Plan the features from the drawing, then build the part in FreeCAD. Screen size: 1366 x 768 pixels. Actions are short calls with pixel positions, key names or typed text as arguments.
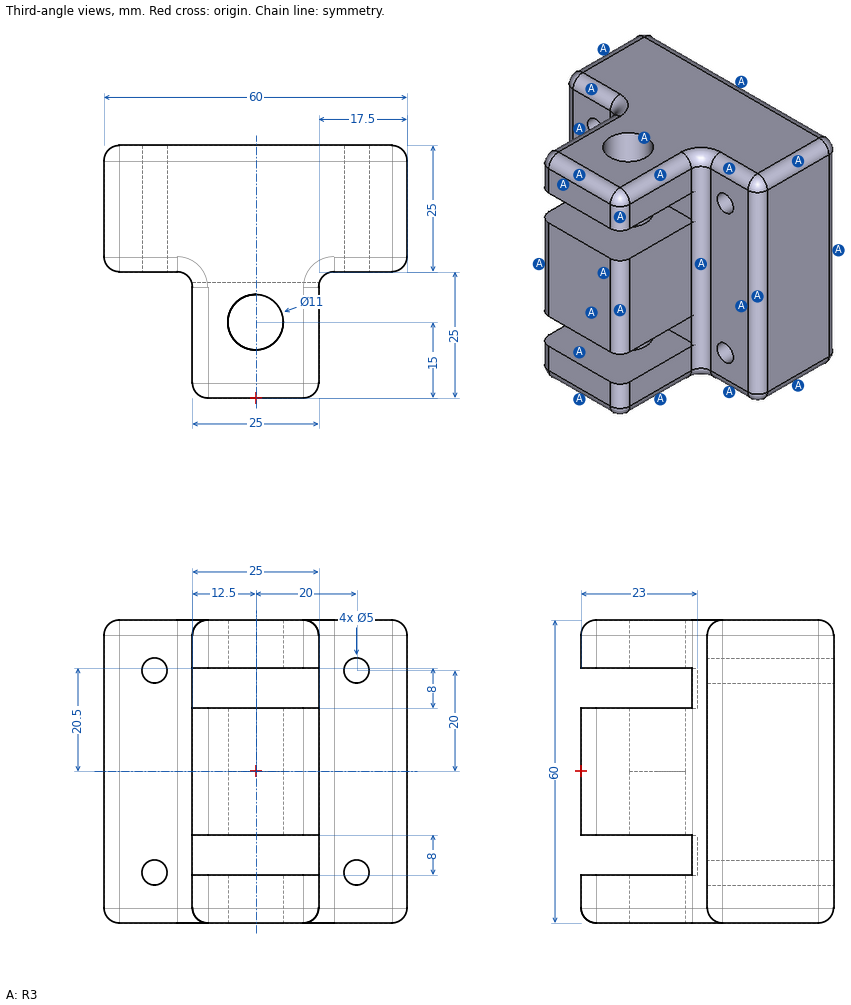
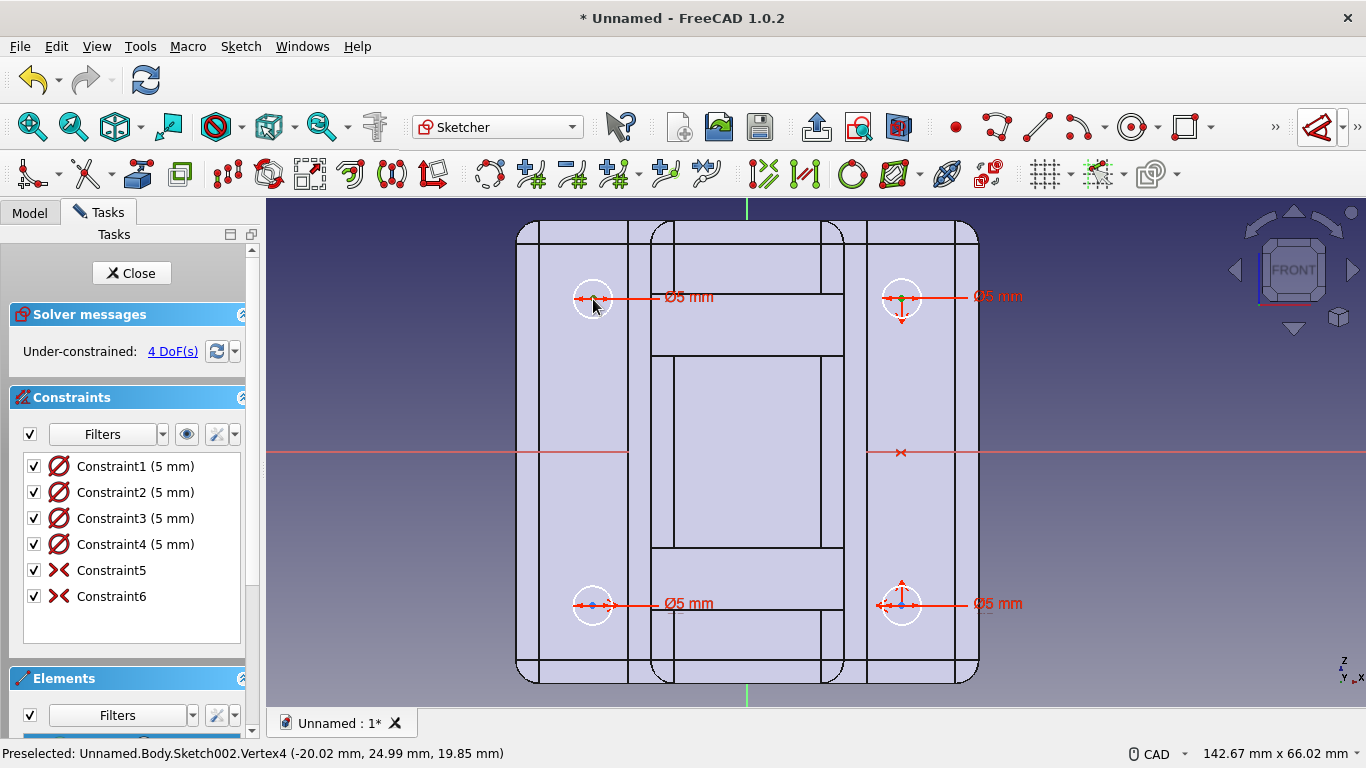
click(747, 647)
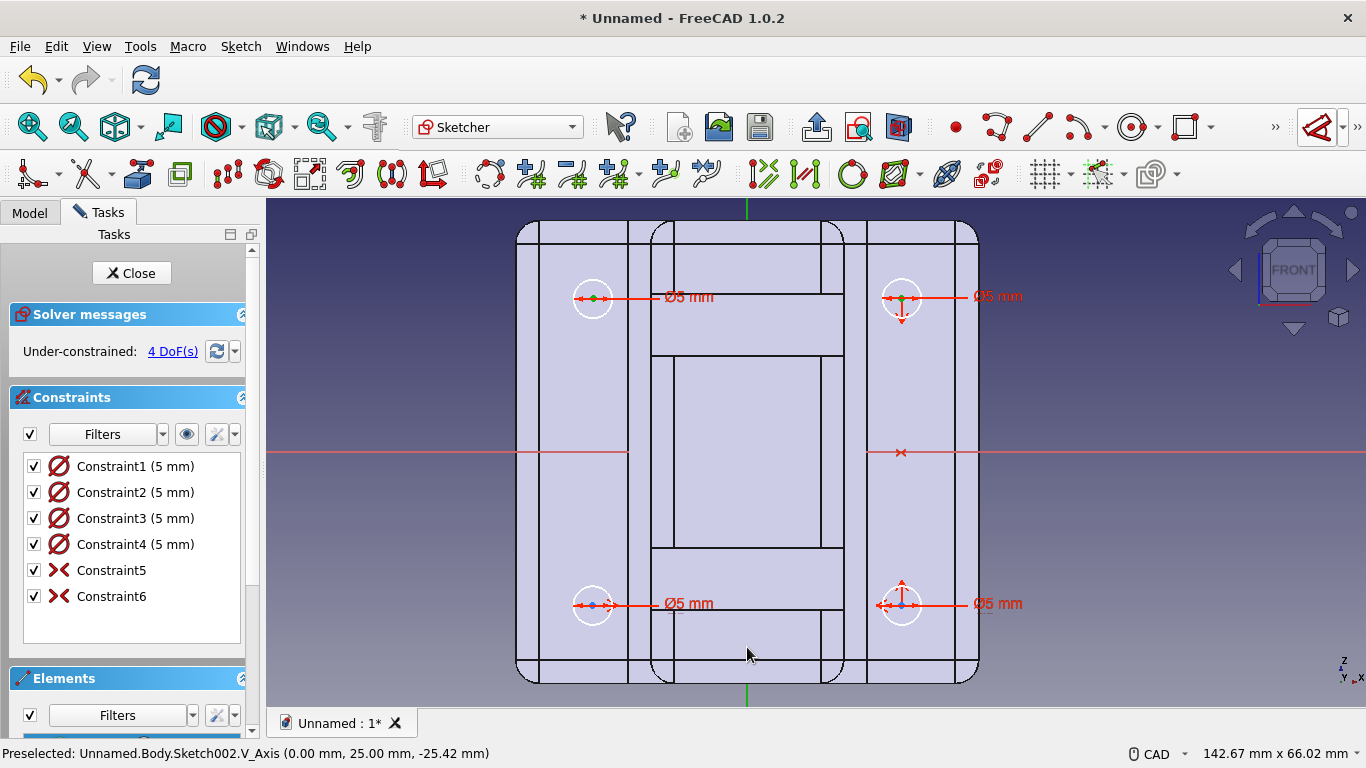
key(s)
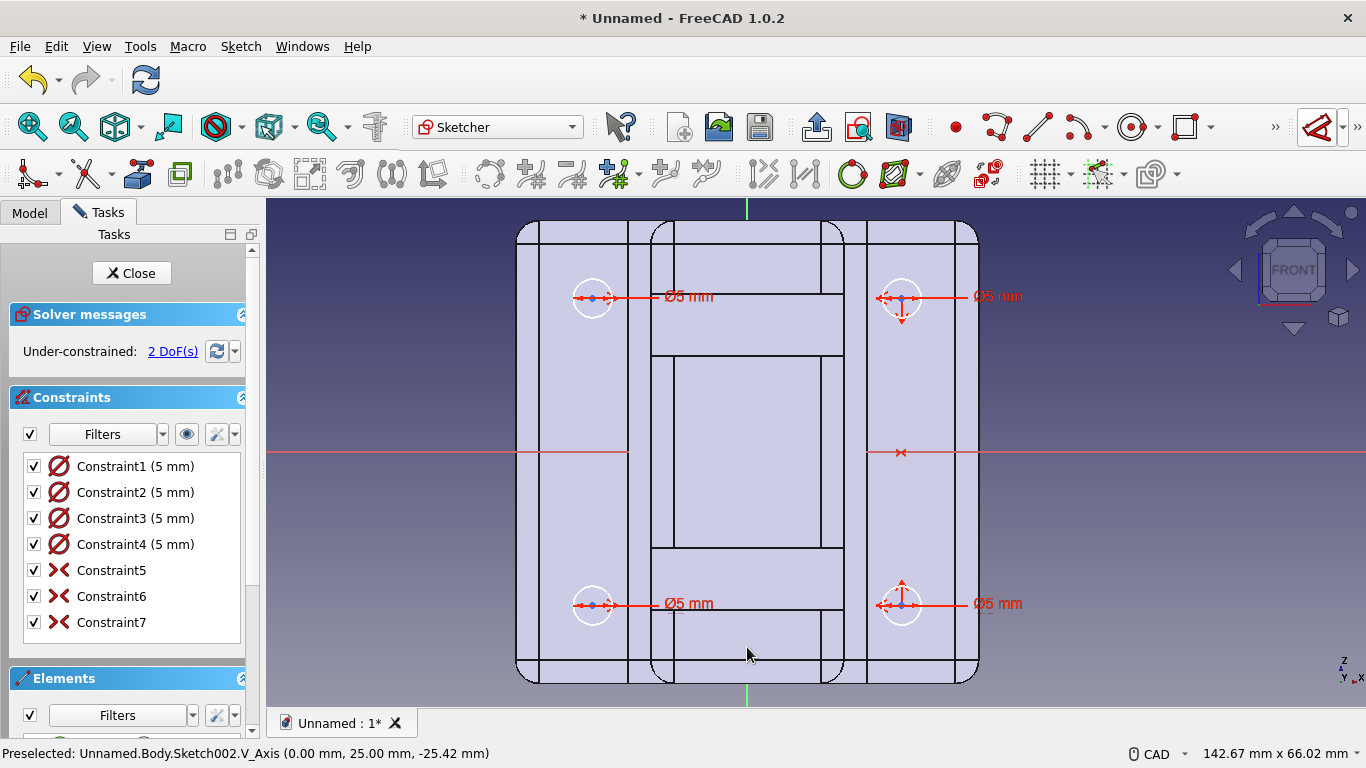
click(902, 298)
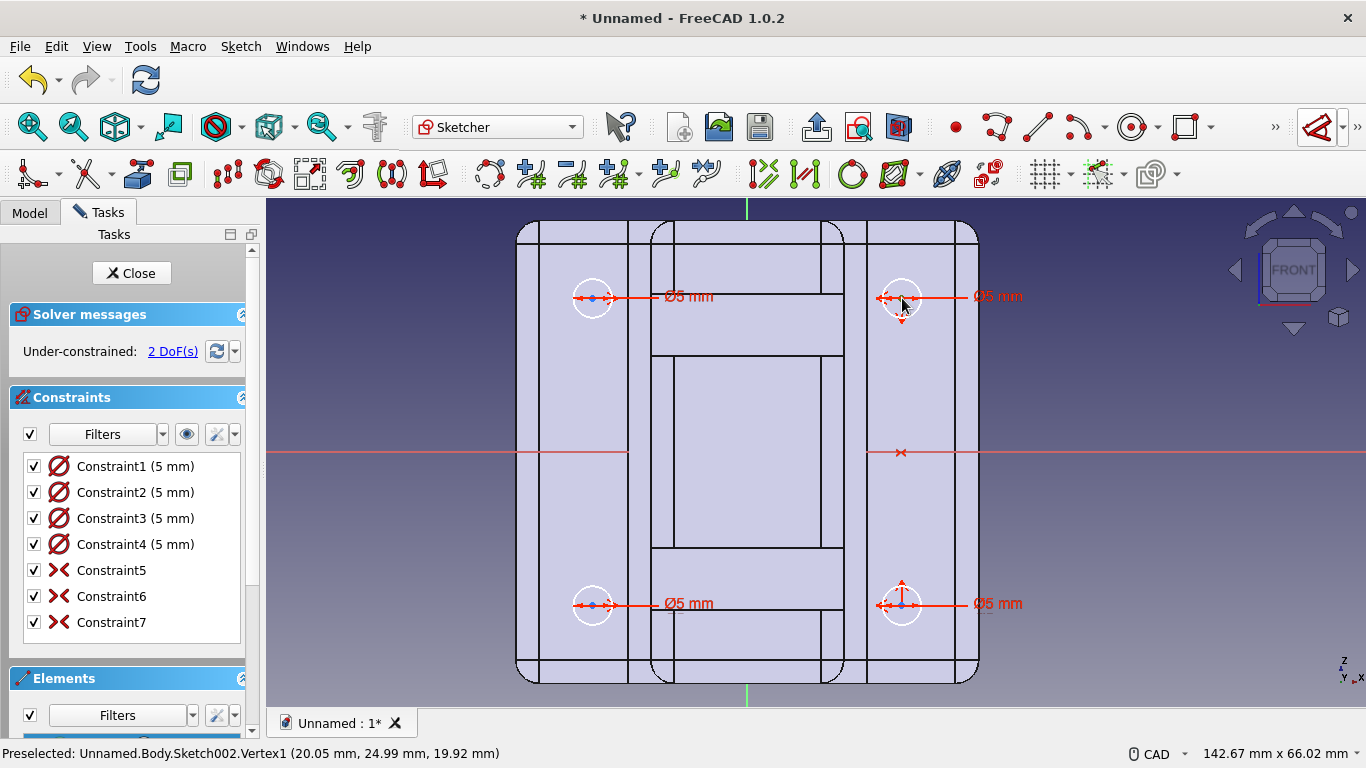
key(l)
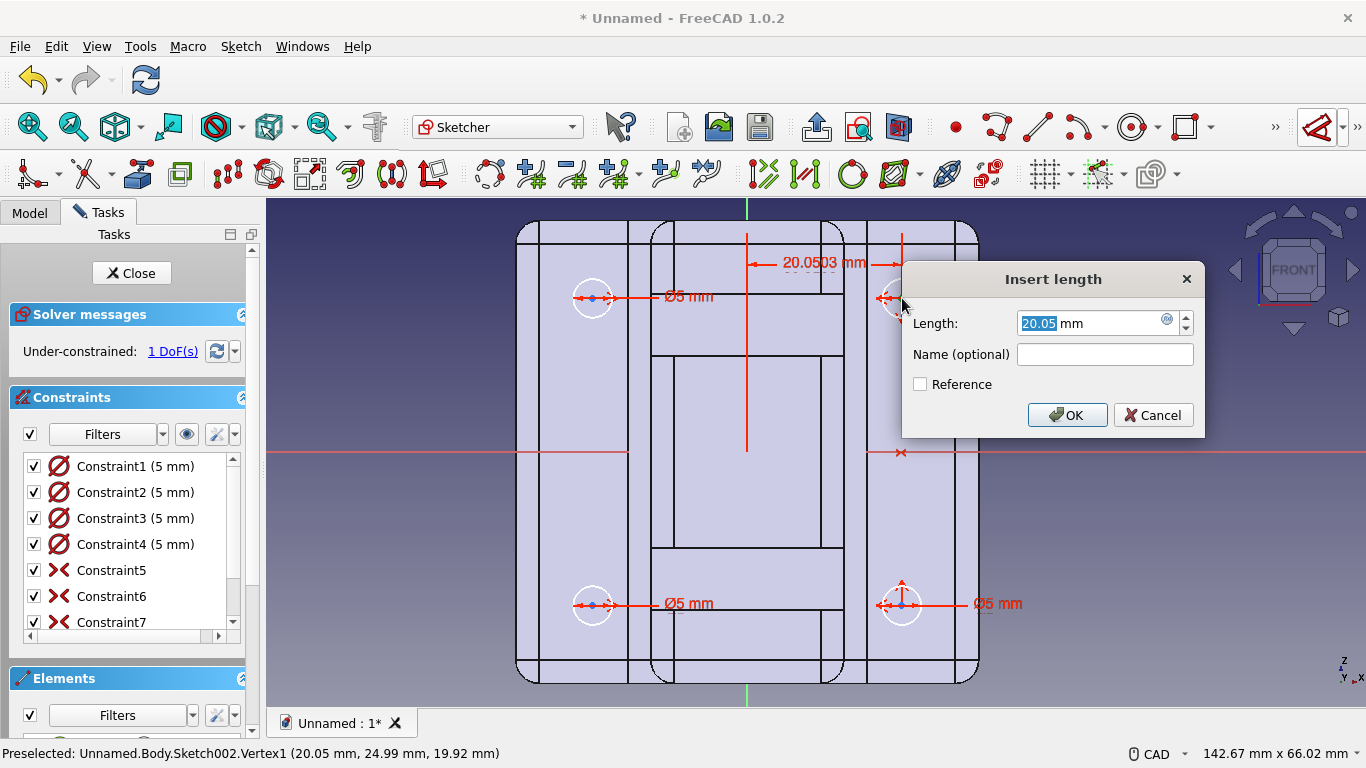
text(20)
key(Return)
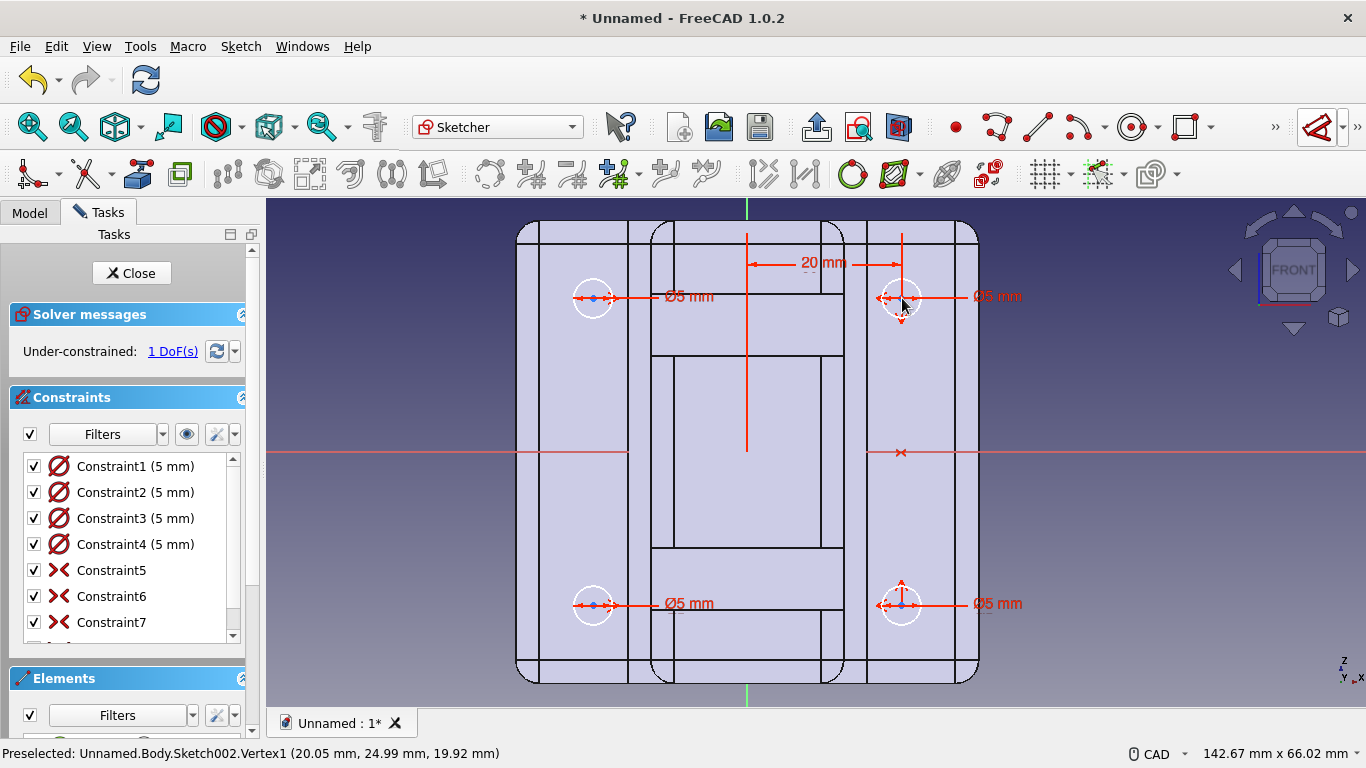
click(902, 298)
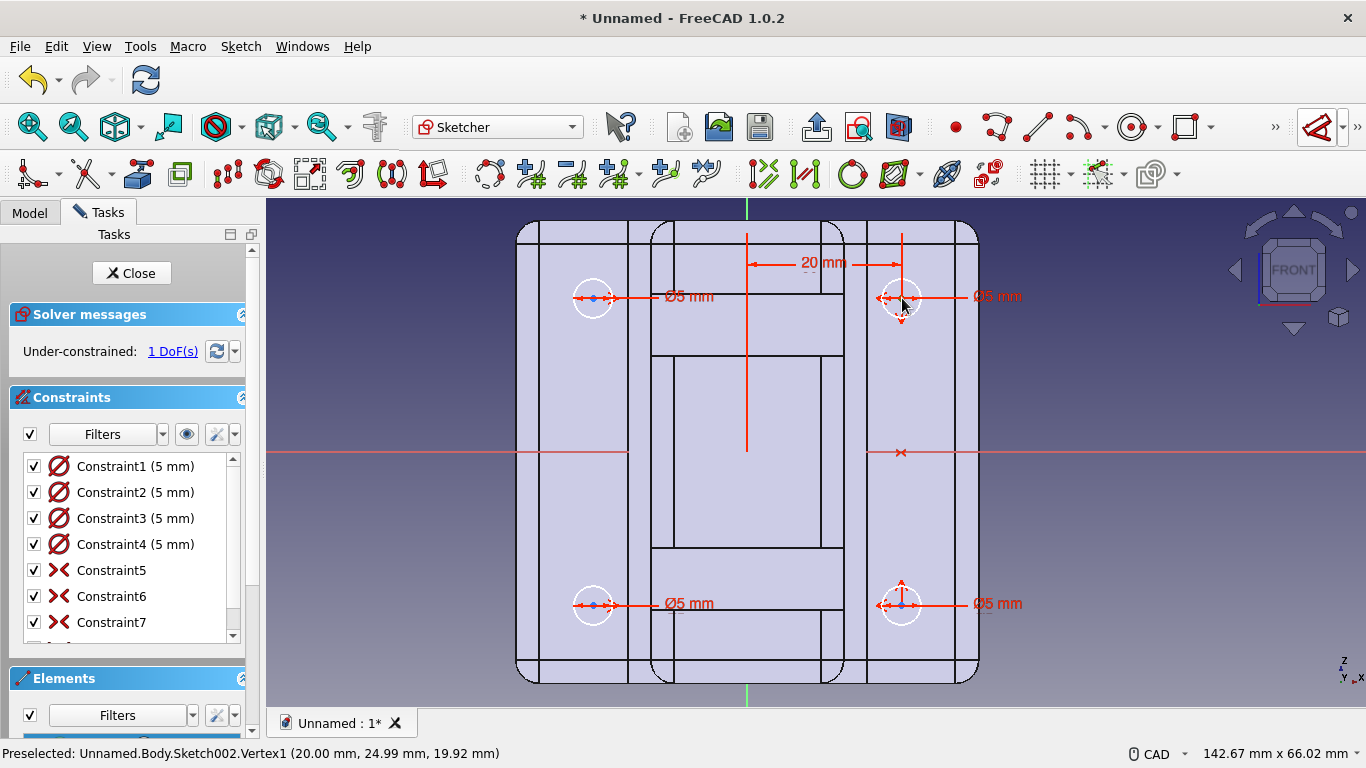
click(1342, 128)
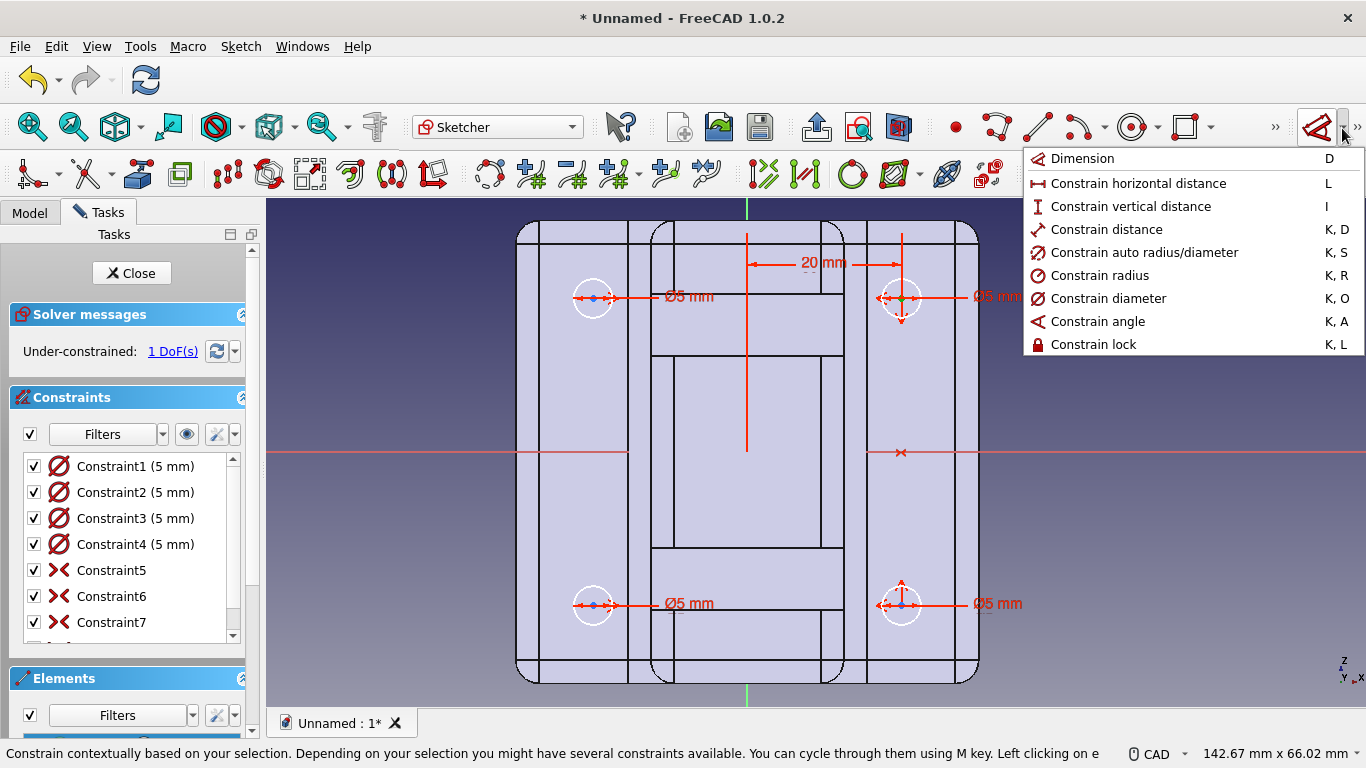
click(1194, 206)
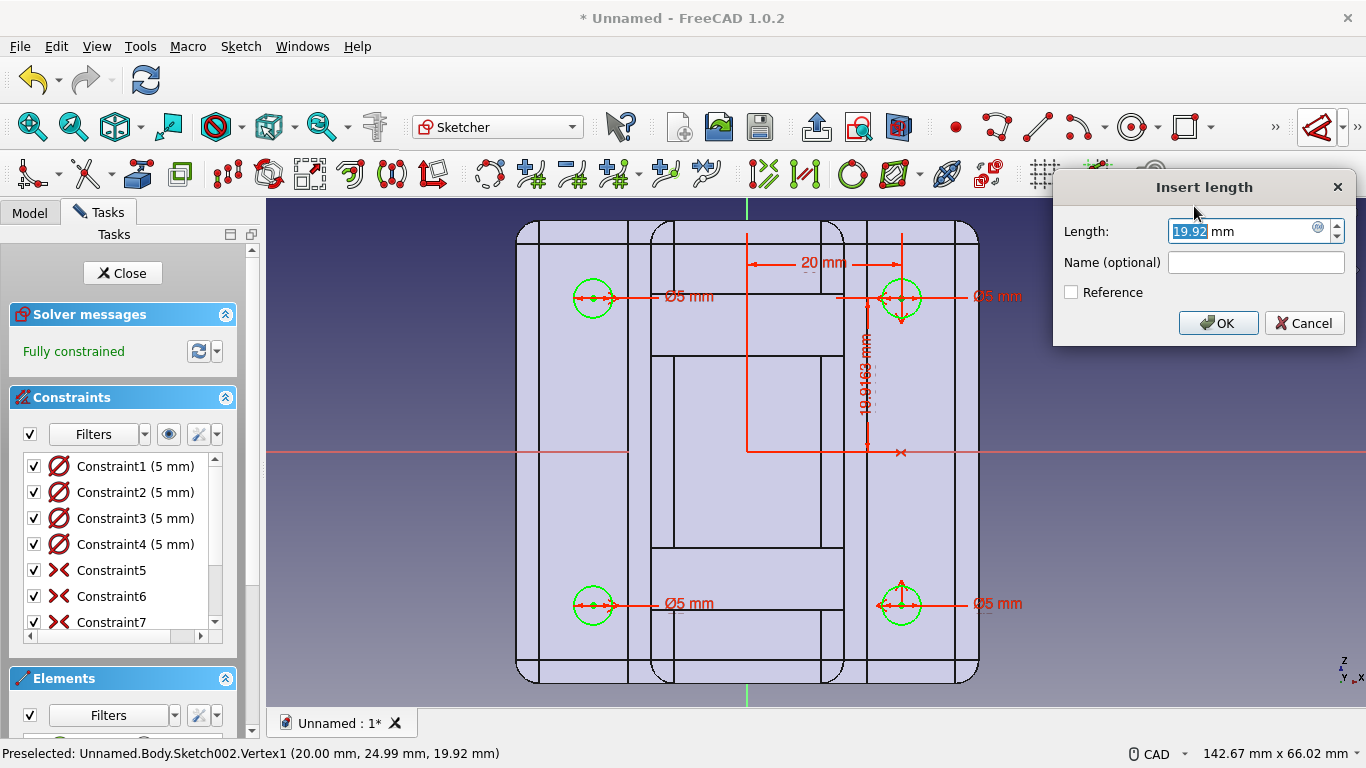
text(20)
key(Return)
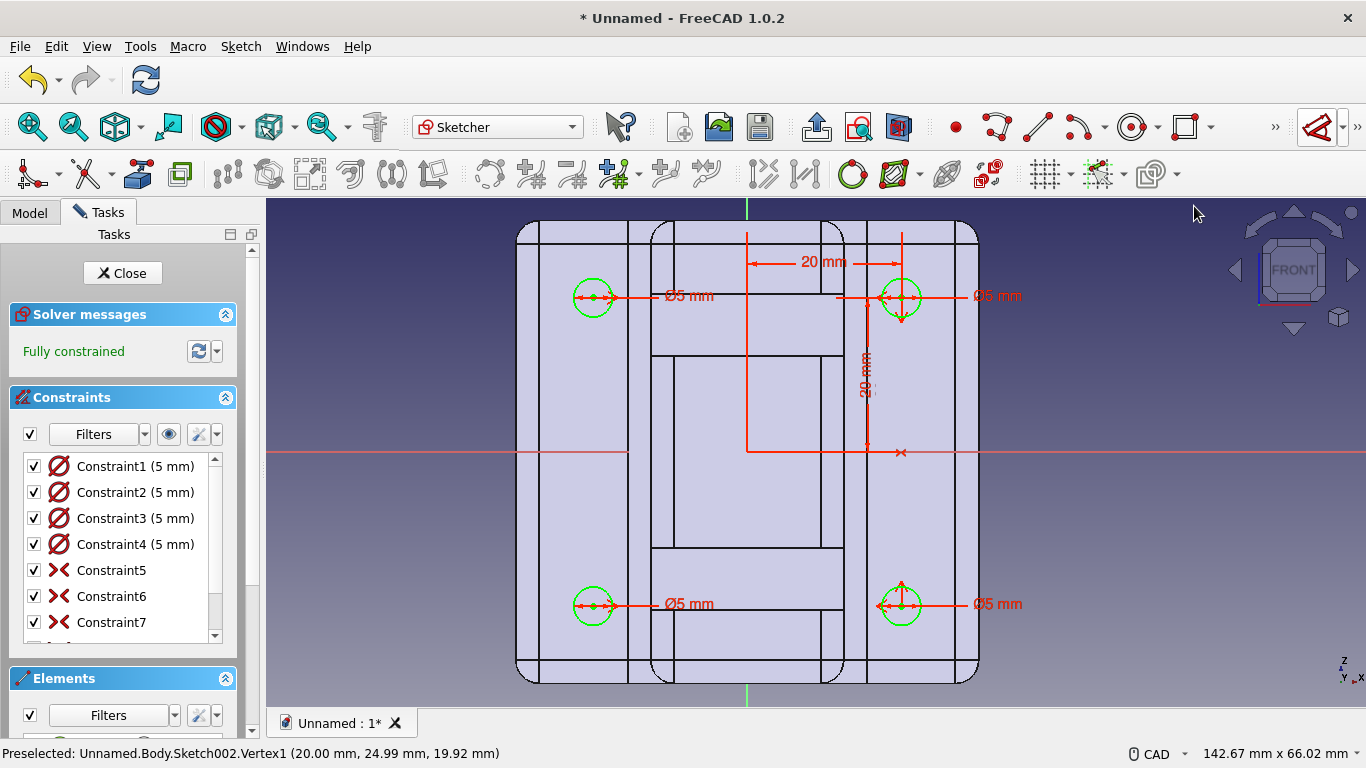
click(123, 273)